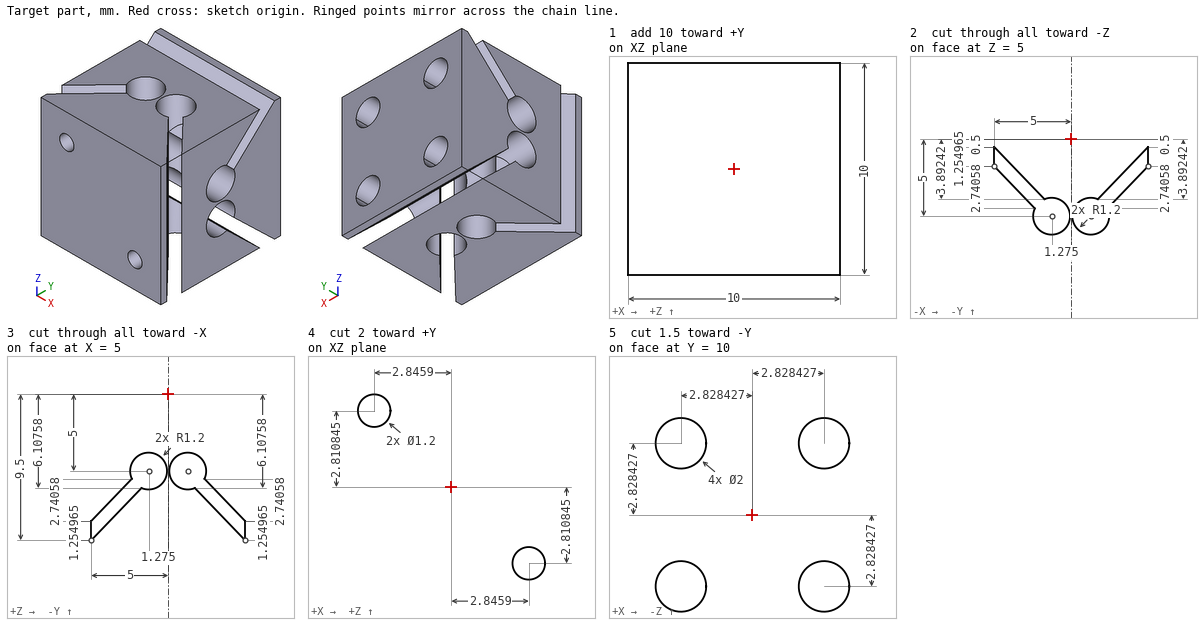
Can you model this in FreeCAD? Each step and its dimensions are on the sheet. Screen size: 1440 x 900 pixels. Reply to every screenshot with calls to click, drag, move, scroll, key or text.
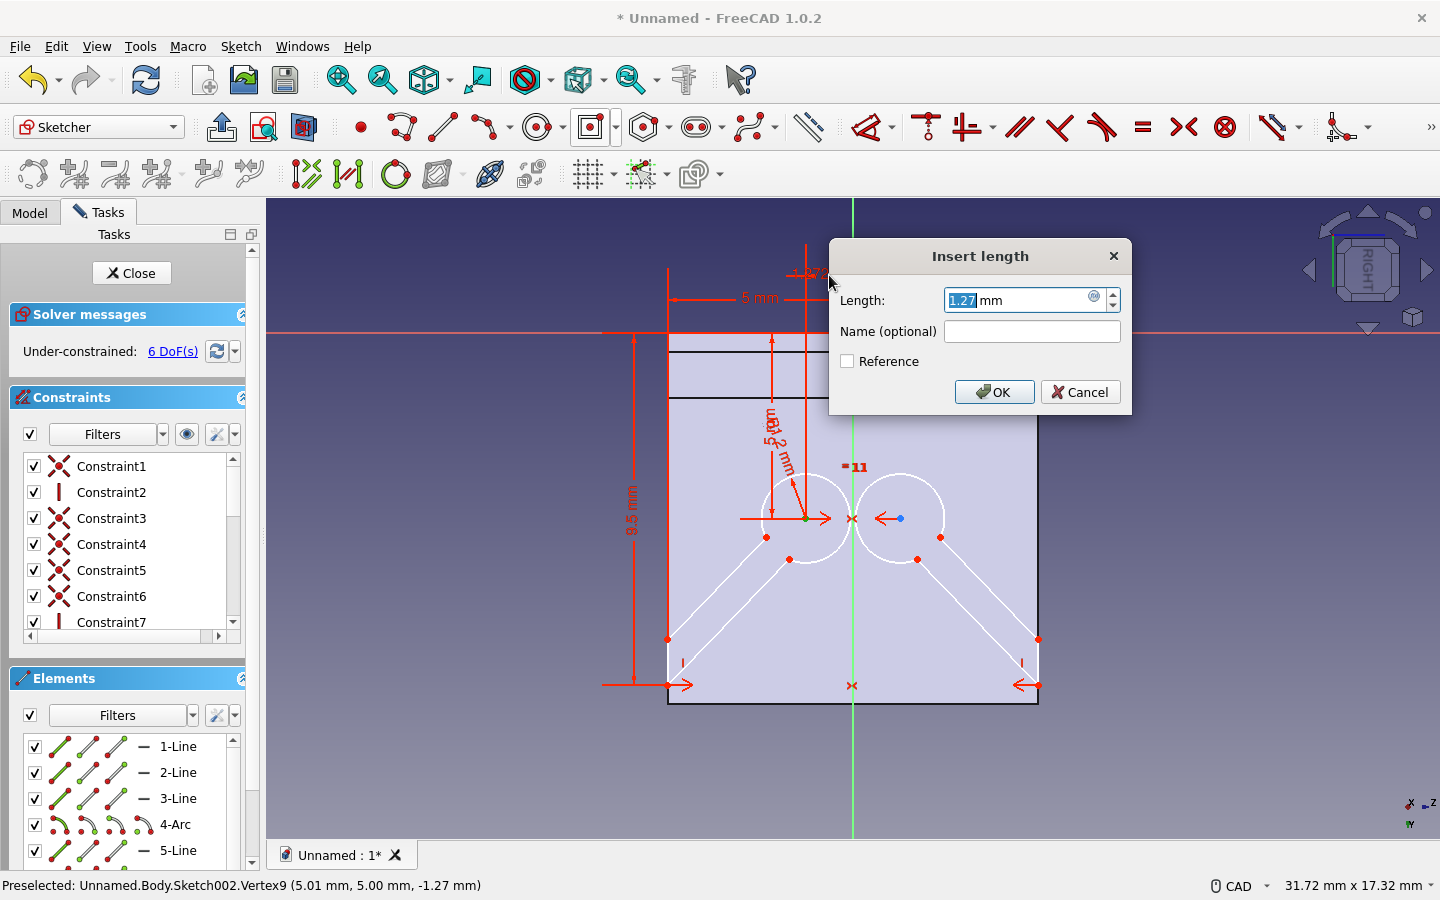
text(1.275)
key(Return)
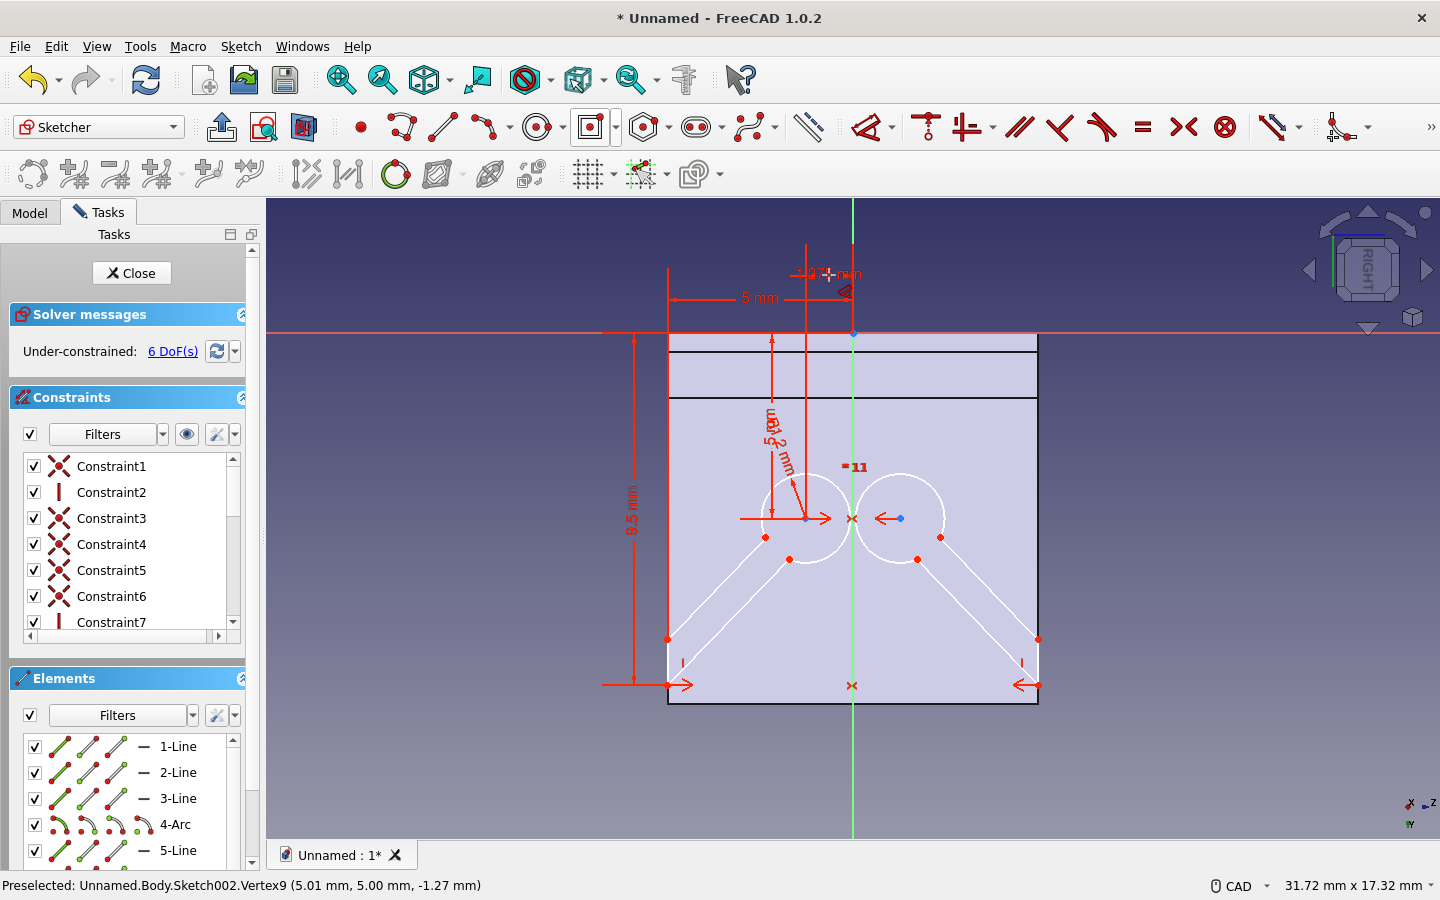
click(668, 654)
click(634, 663)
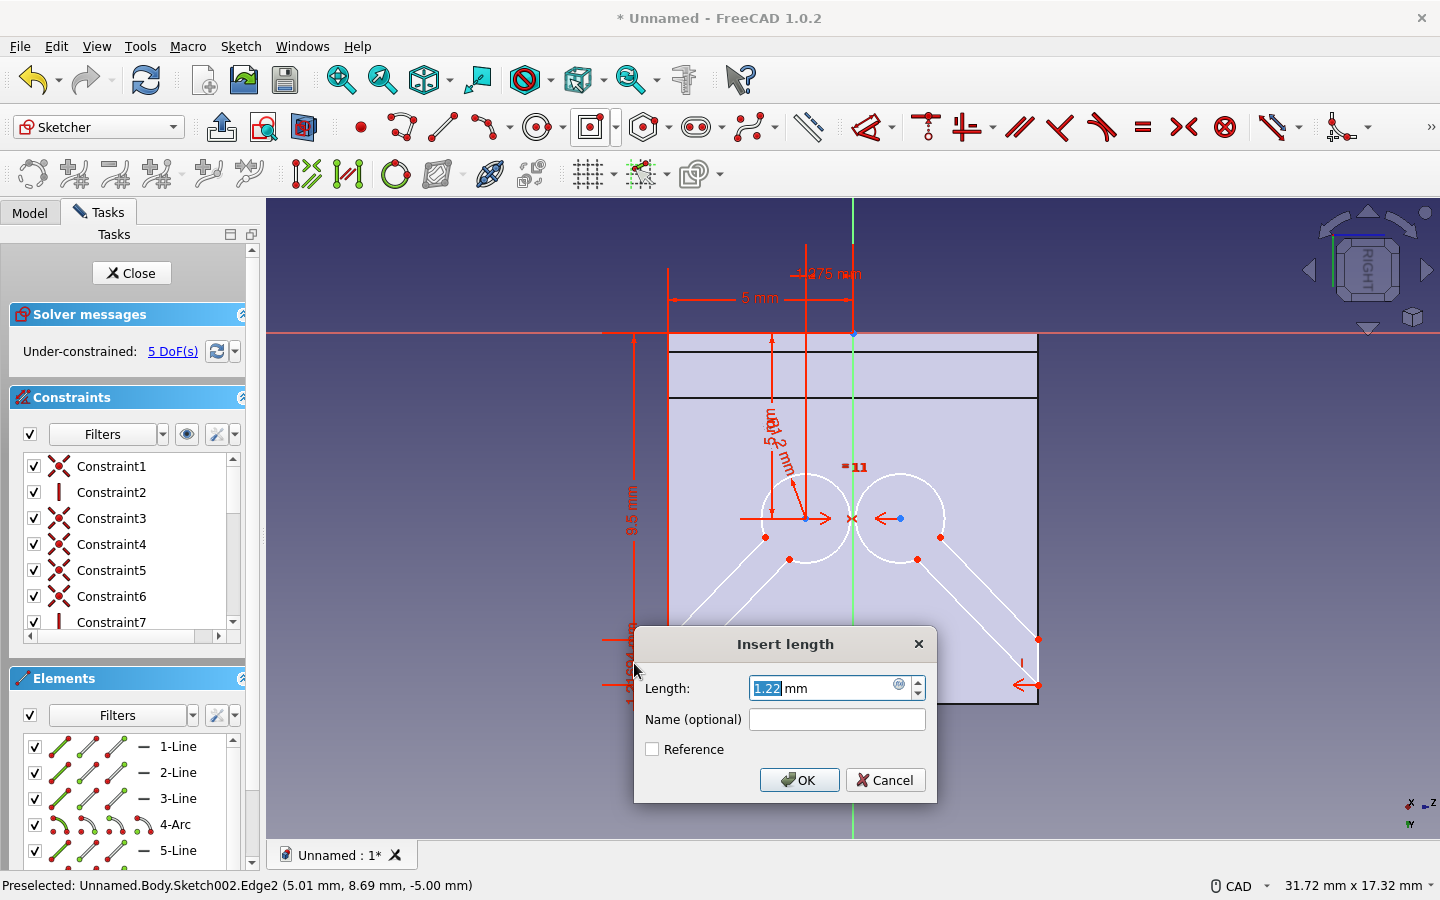
text(1.254965)
key(Return)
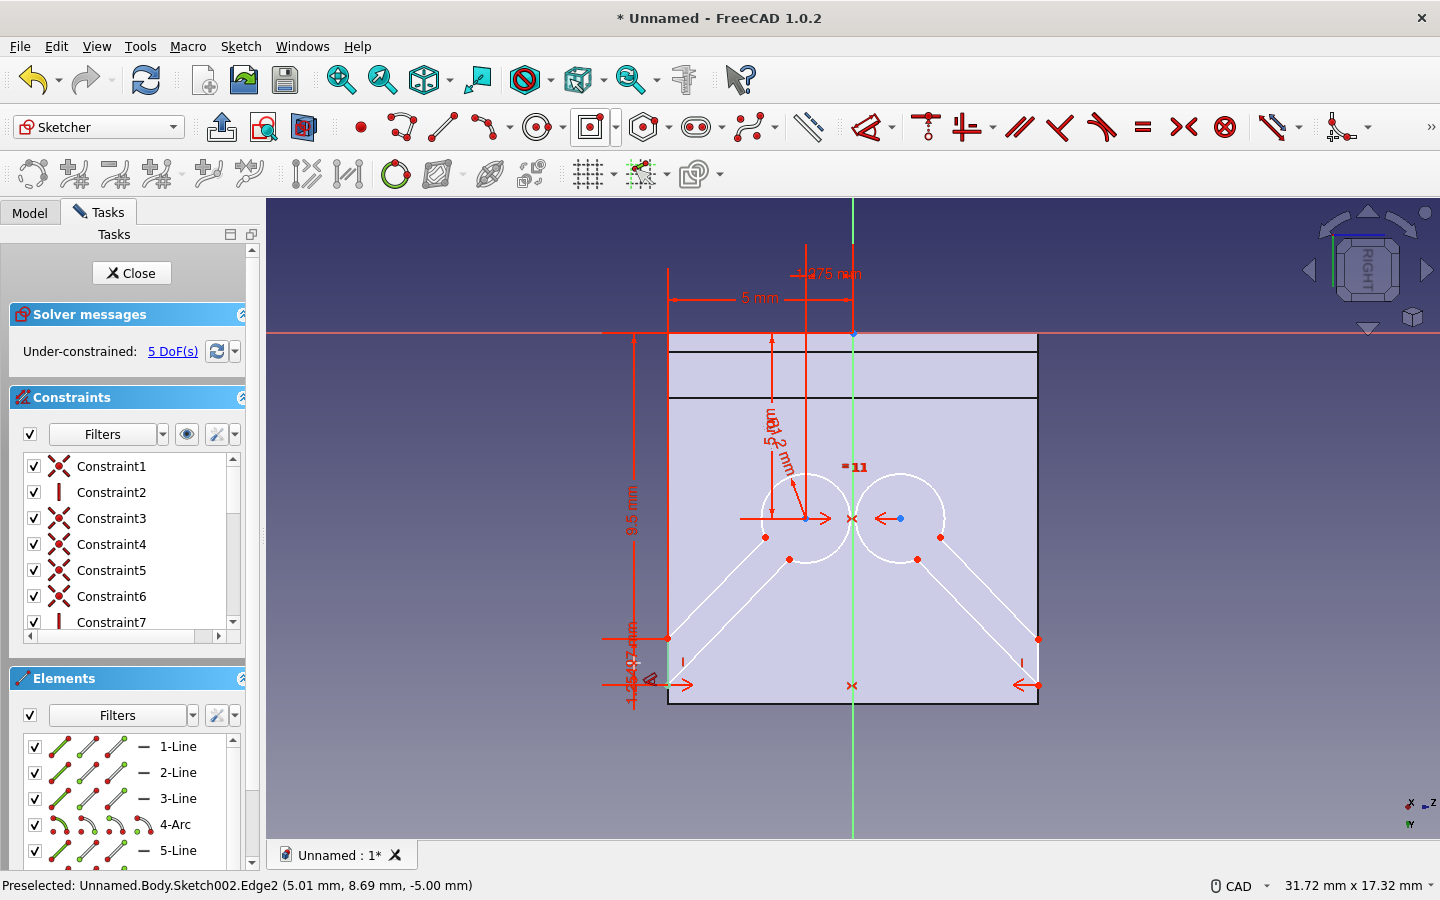
scroll(1038, 672, up, 2)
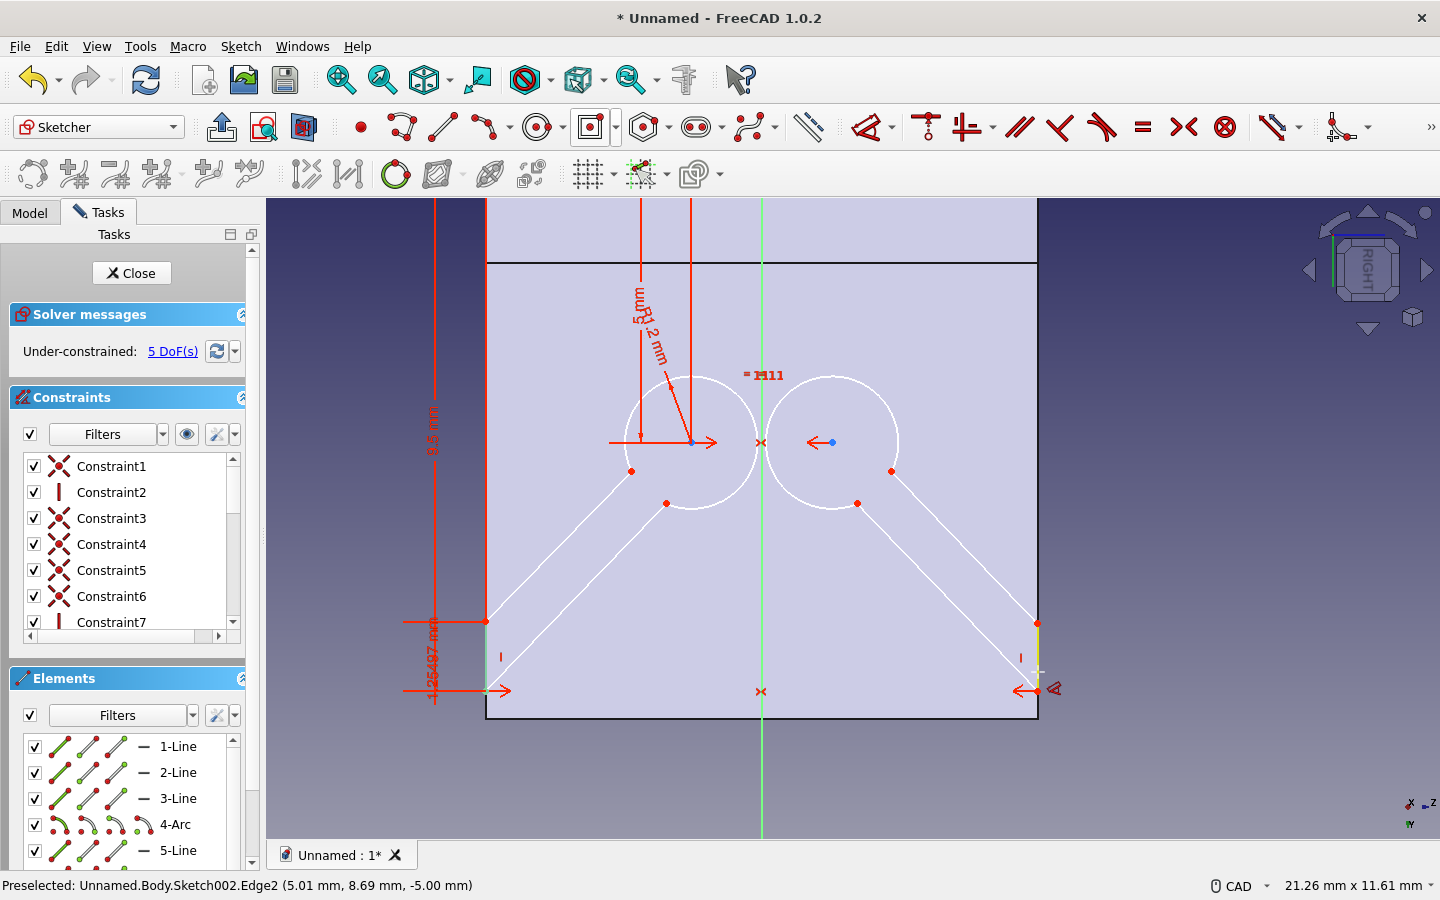
click(1038, 671)
click(1072, 657)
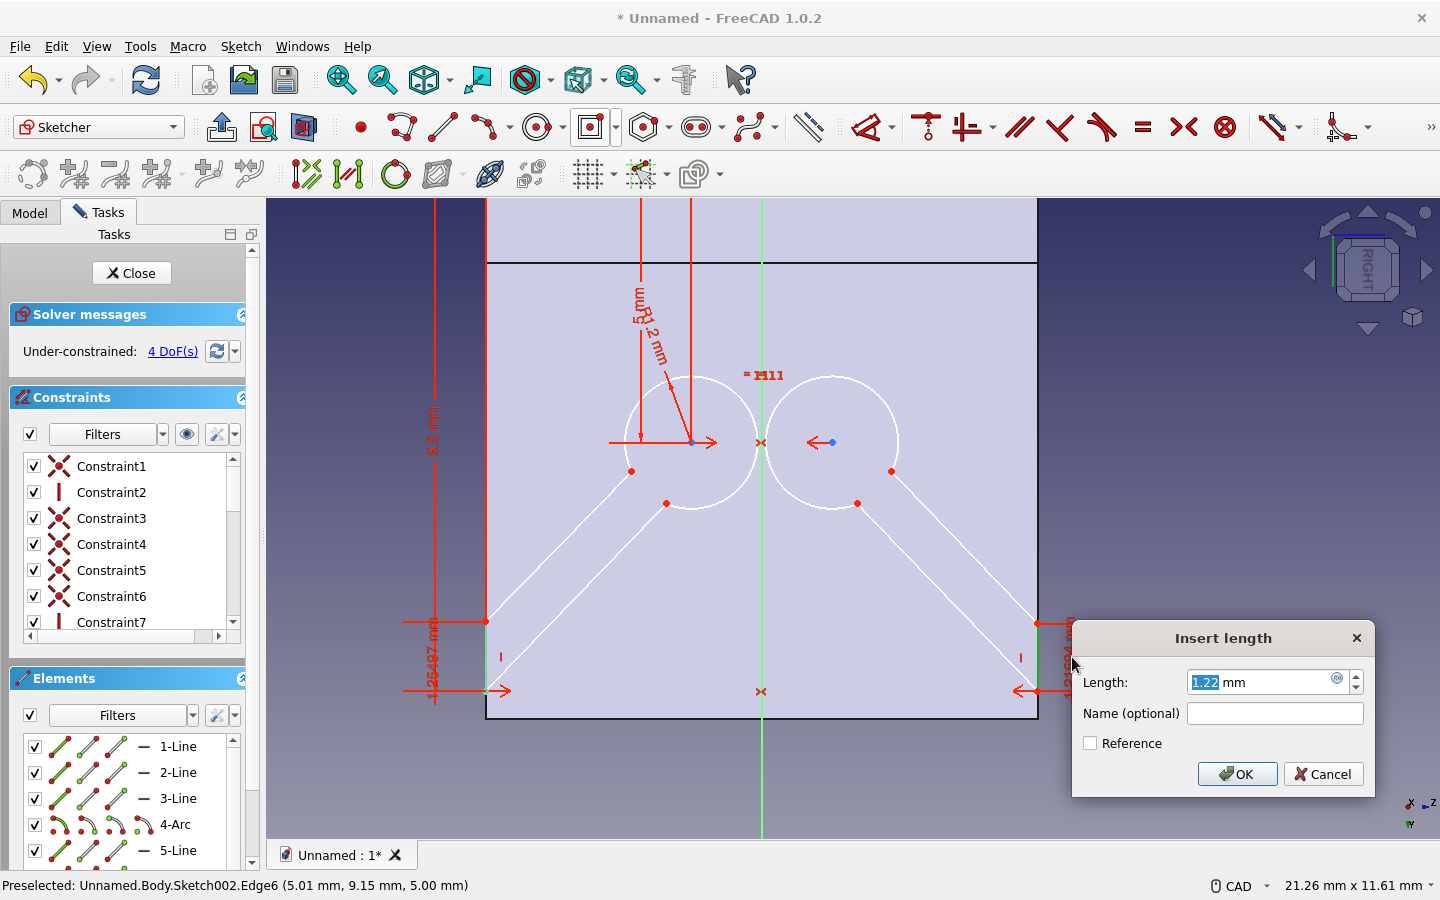
text(1.254965)
key(Return)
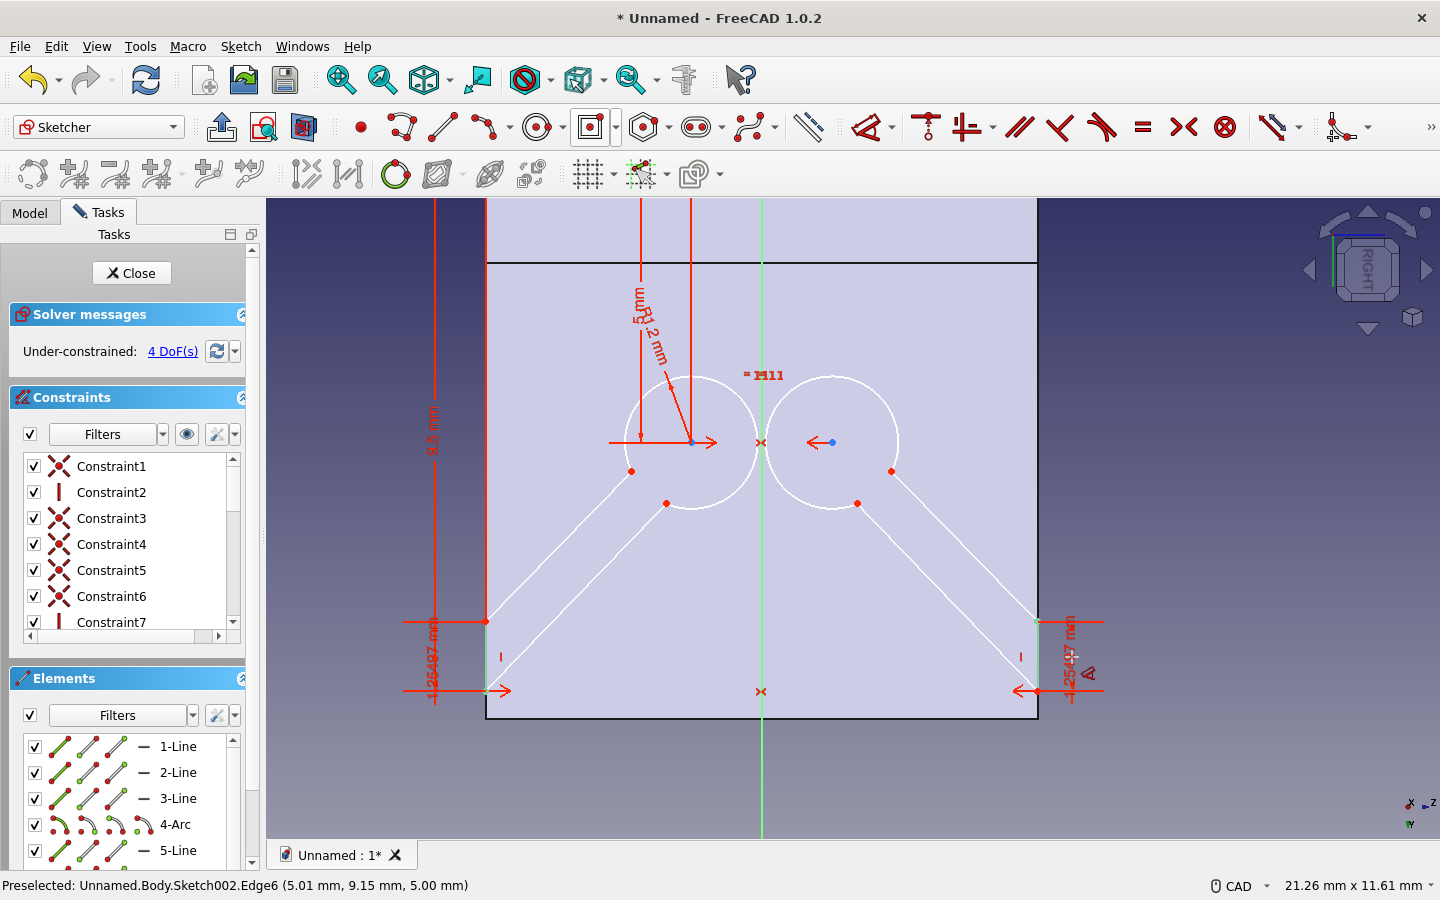
click(666, 504)
click(632, 365)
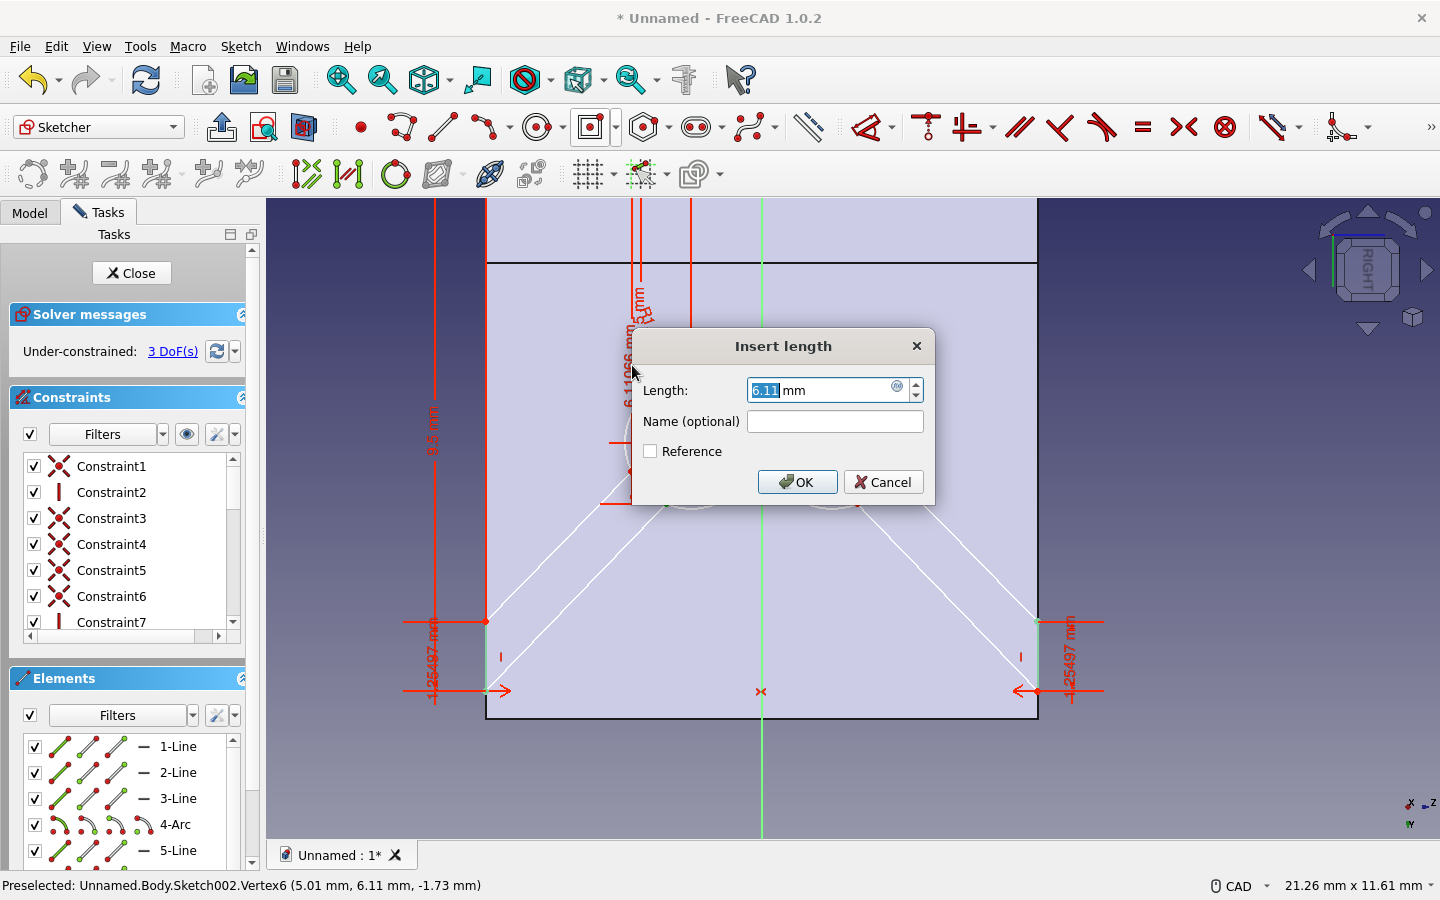
text(6.10758)
key(Return)